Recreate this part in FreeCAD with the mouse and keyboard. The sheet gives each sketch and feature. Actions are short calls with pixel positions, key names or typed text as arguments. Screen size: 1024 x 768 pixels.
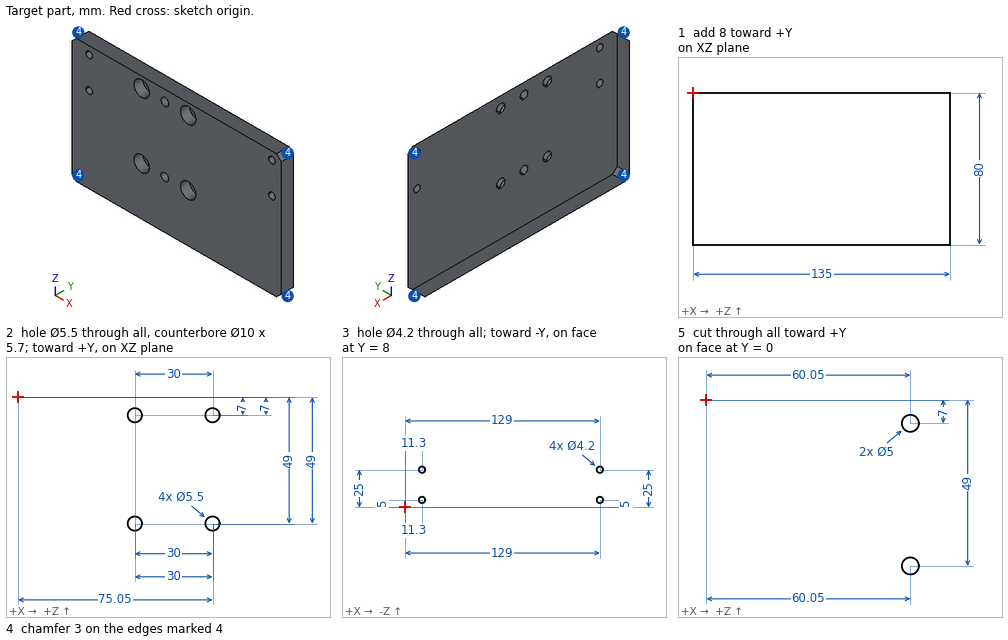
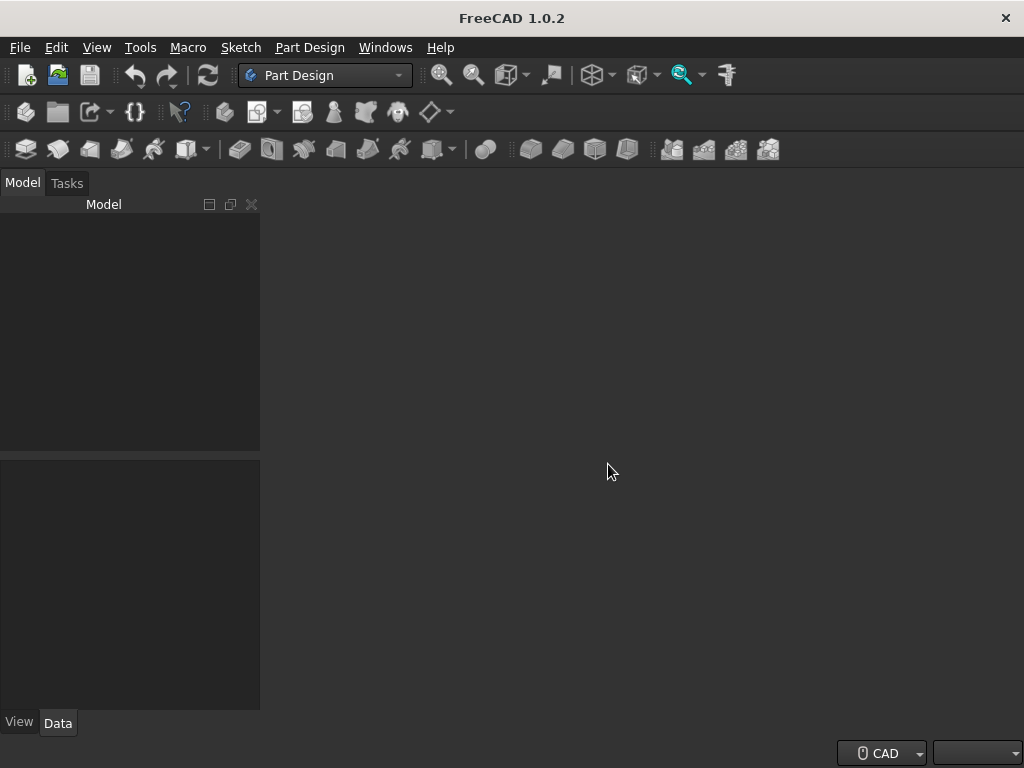
key(ctrl+n)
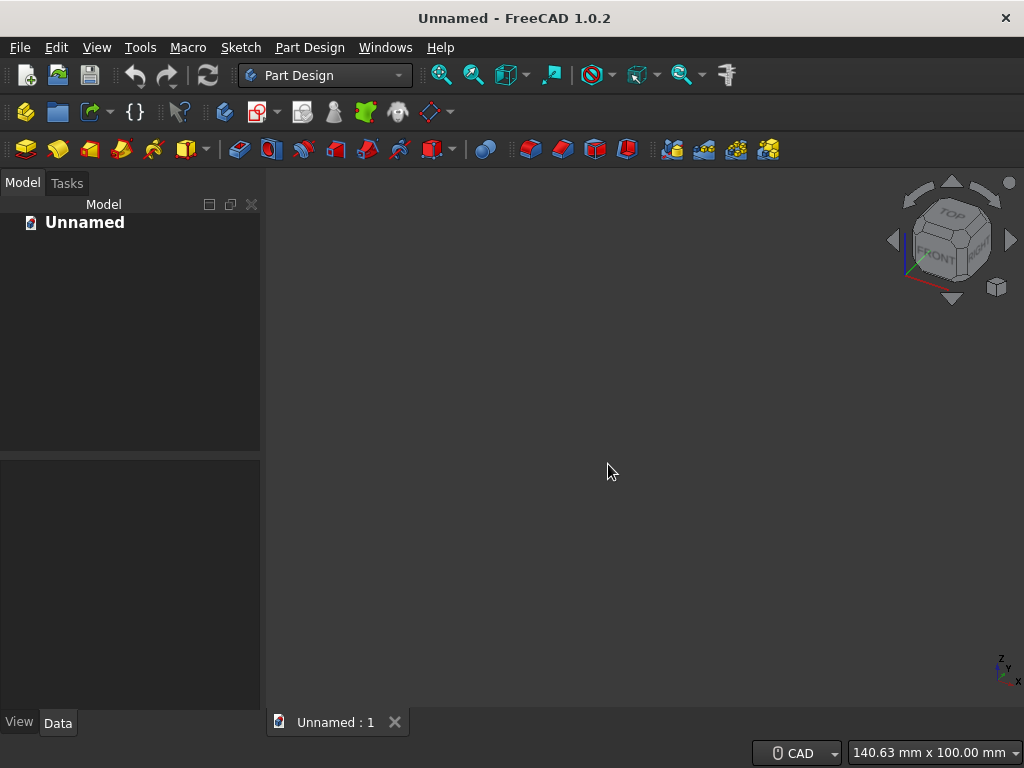
click(258, 112)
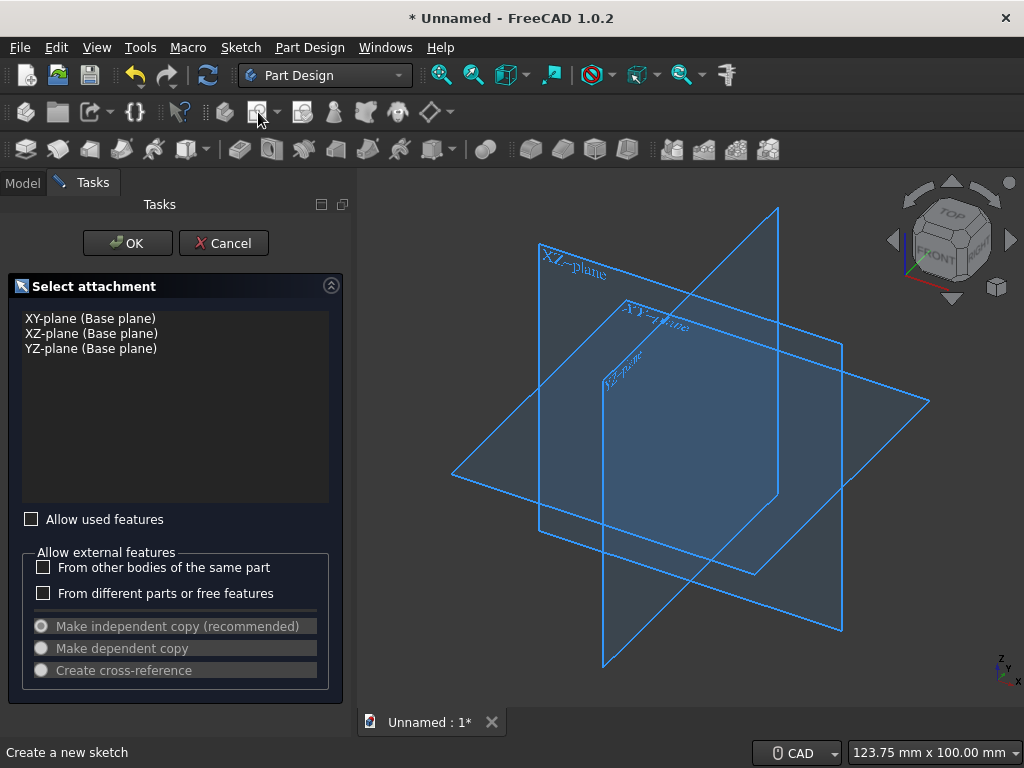
click(82, 334)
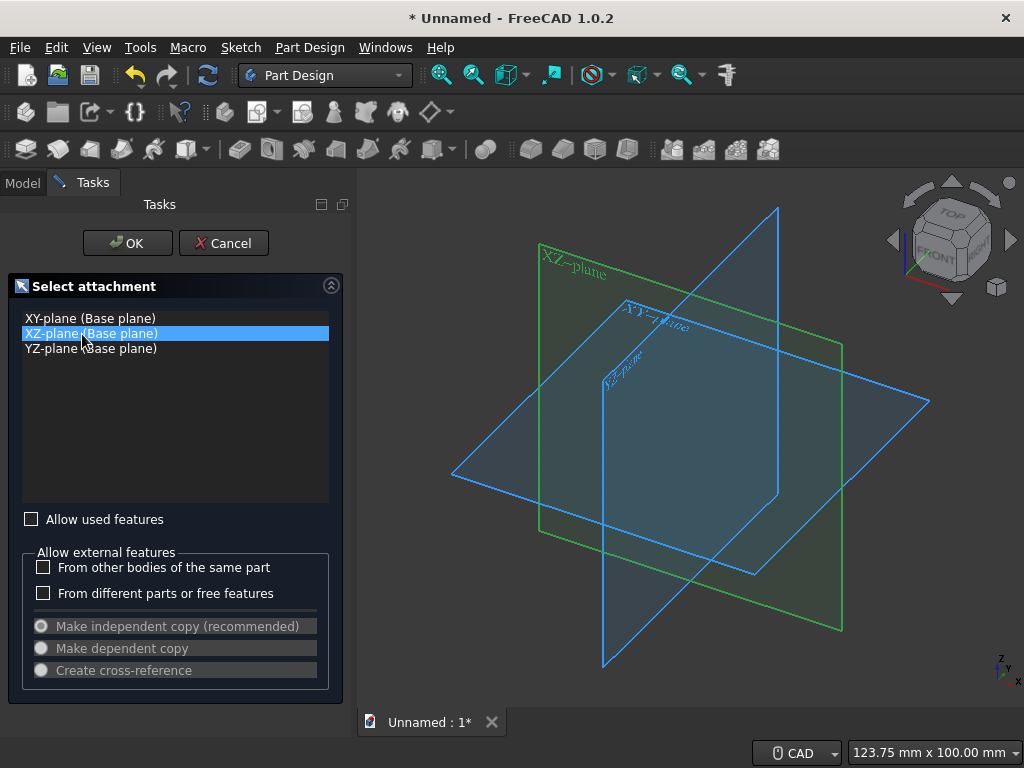
click(128, 243)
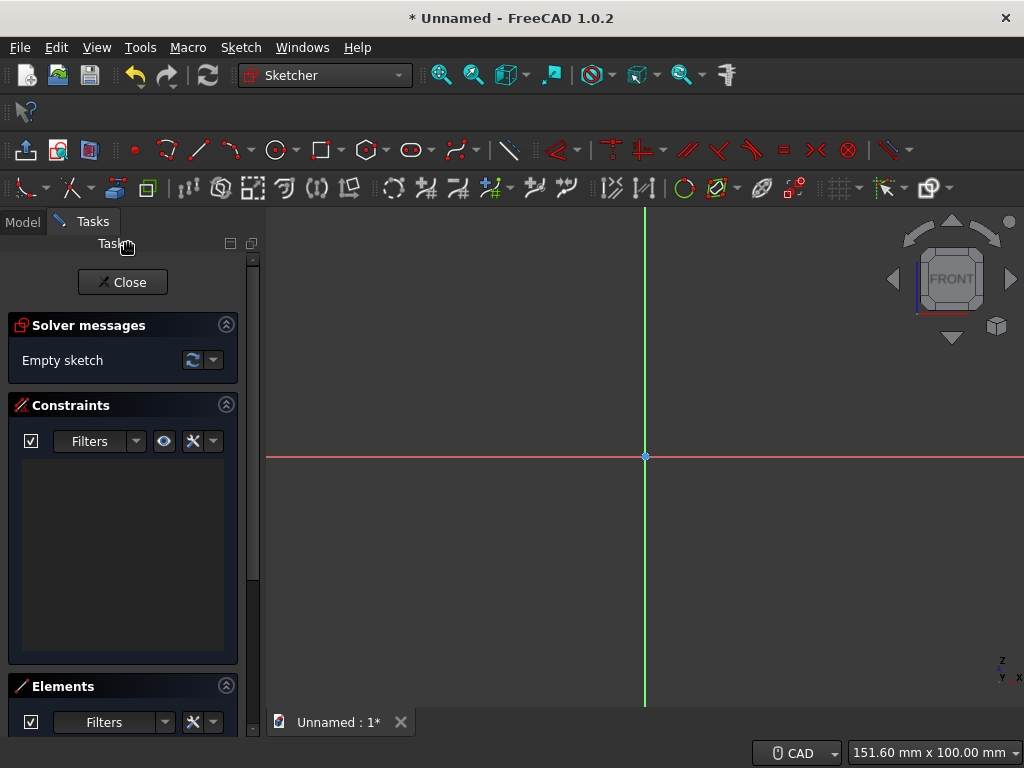
scroll(294, 294, down, 4)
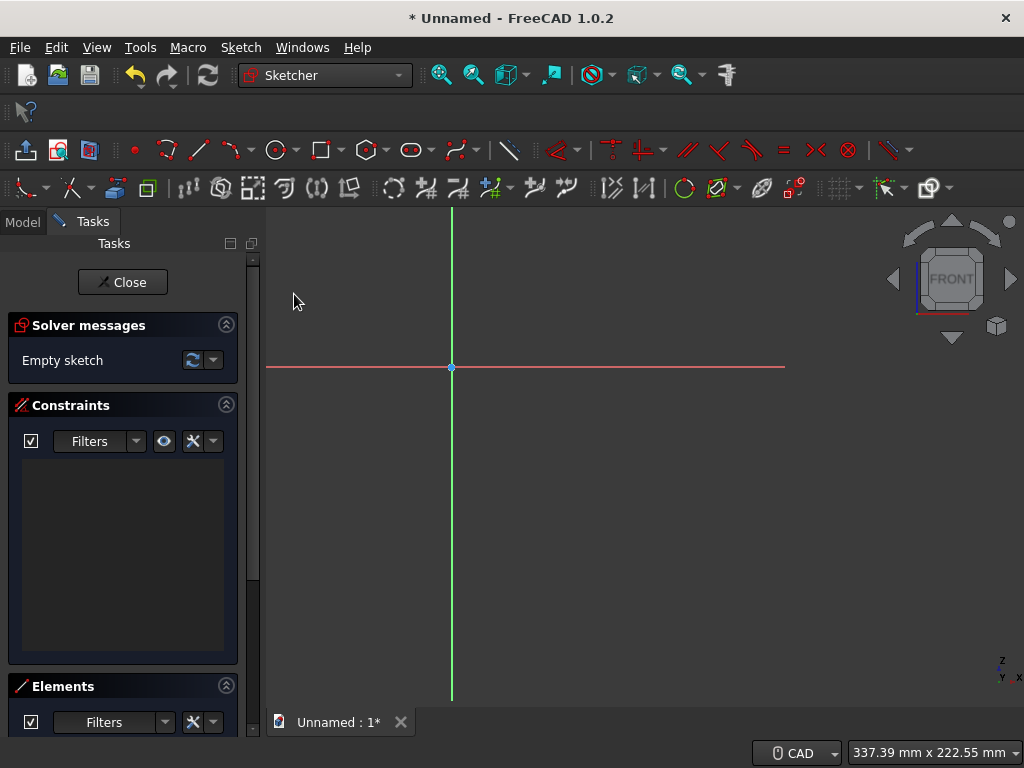
click(322, 150)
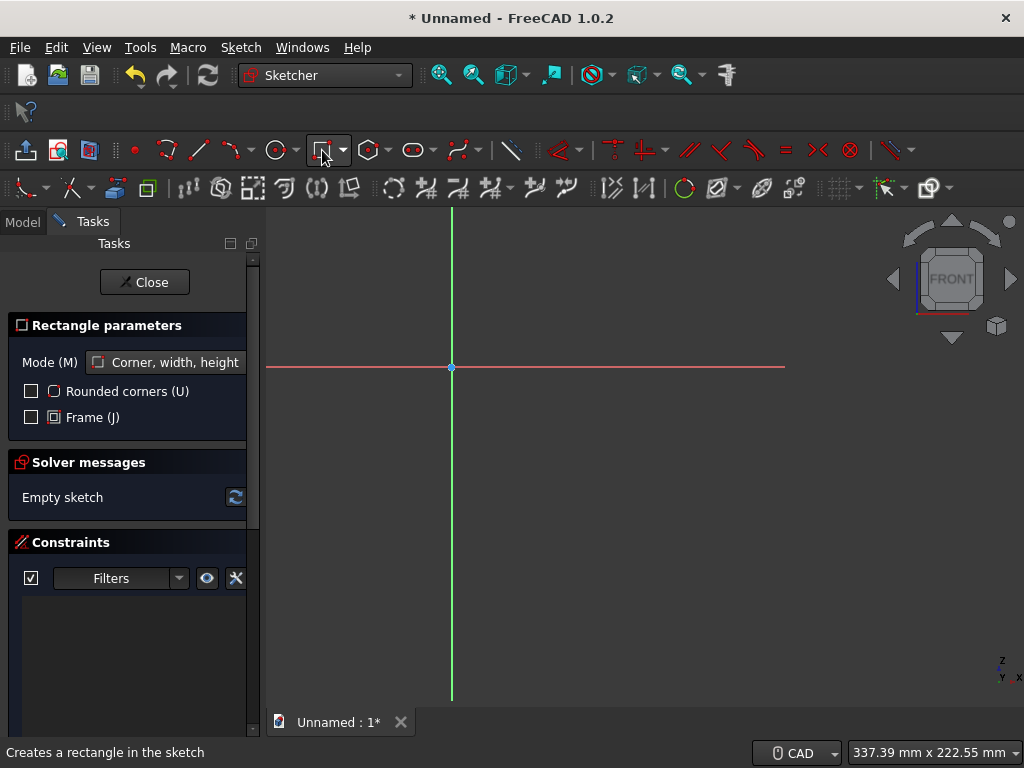
click(452, 367)
move(755, 547)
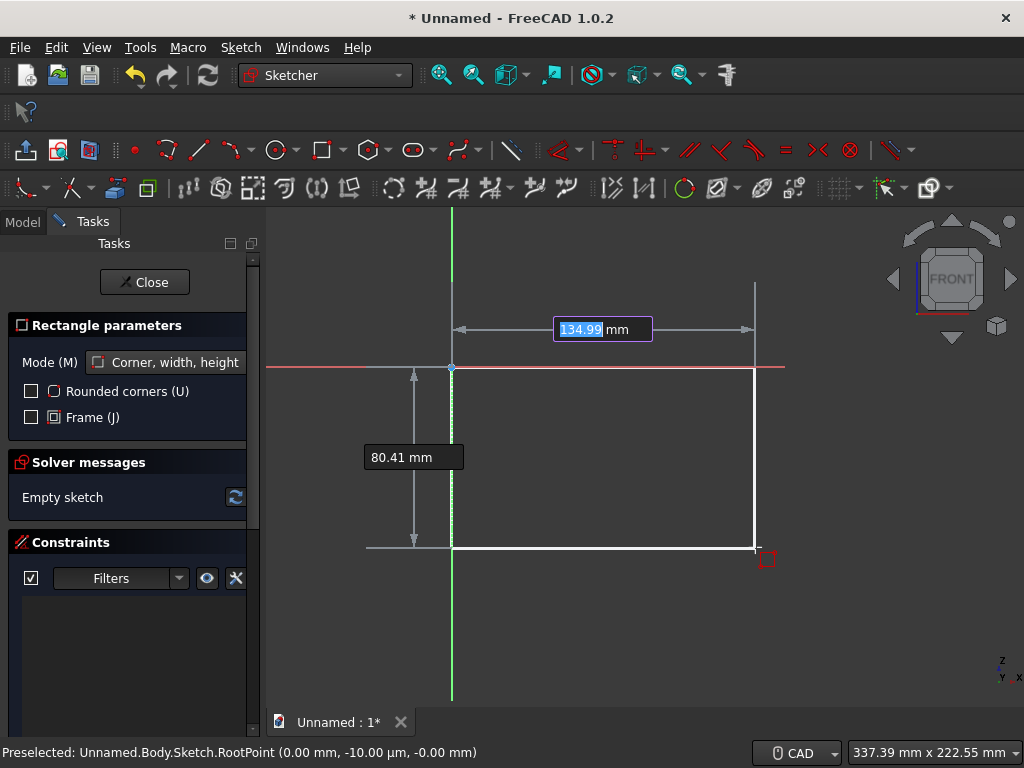
text(135)
key(Tab)
text(80)
key(Return)
key(Escape)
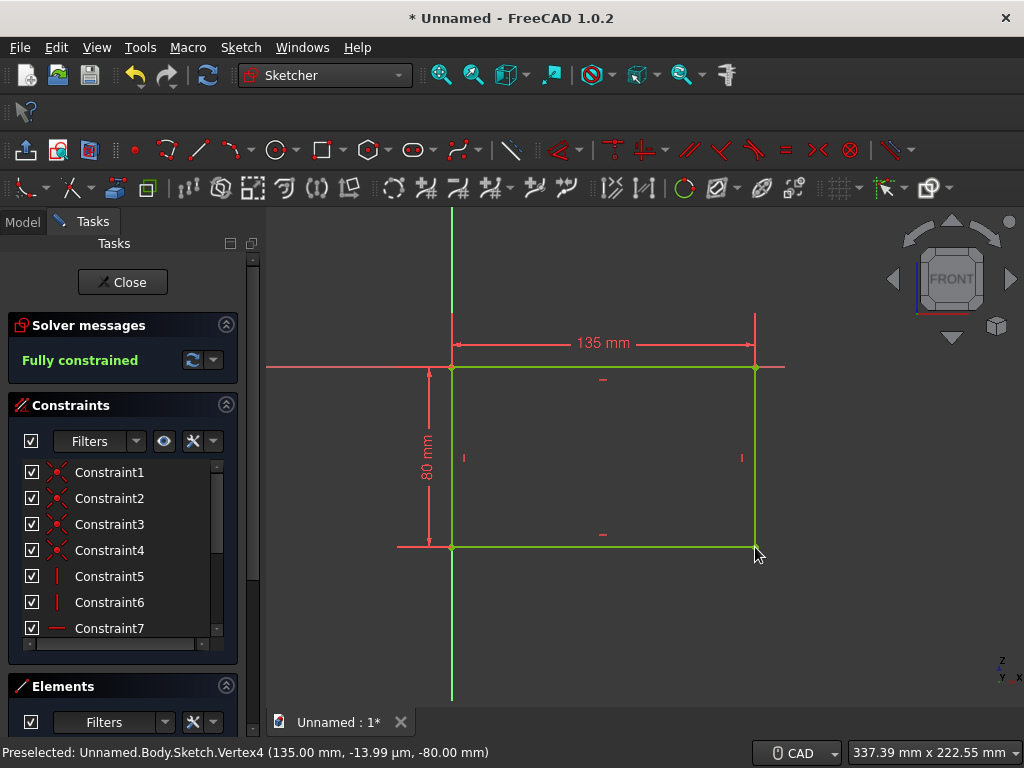
click(123, 282)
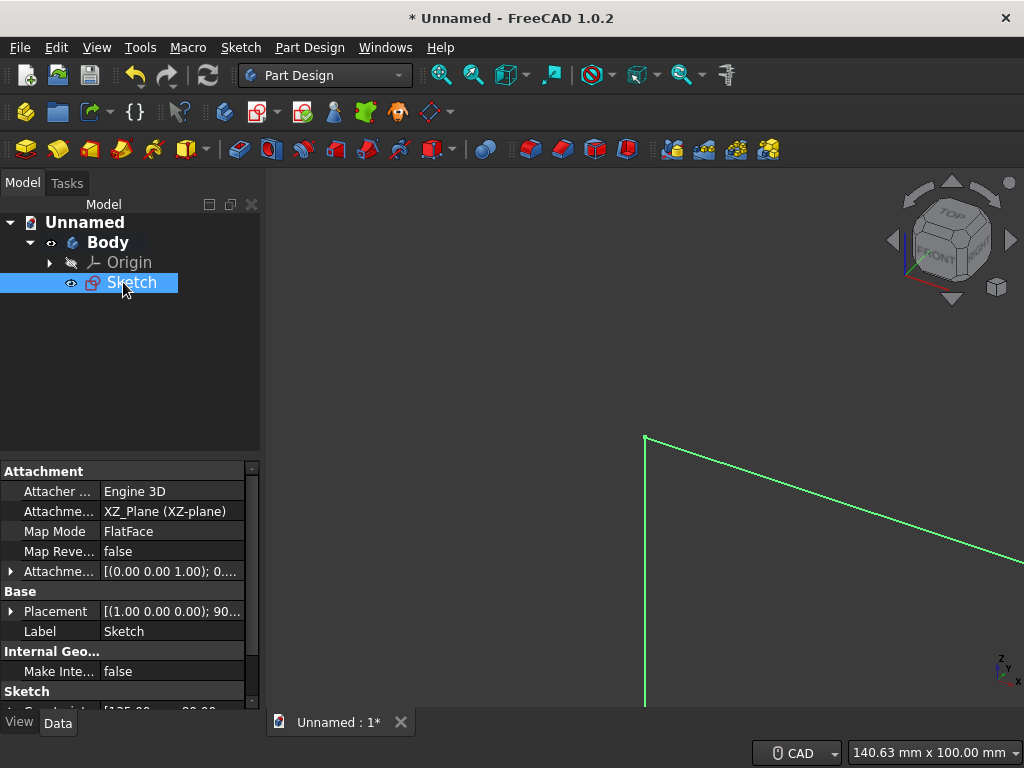
click(26, 150)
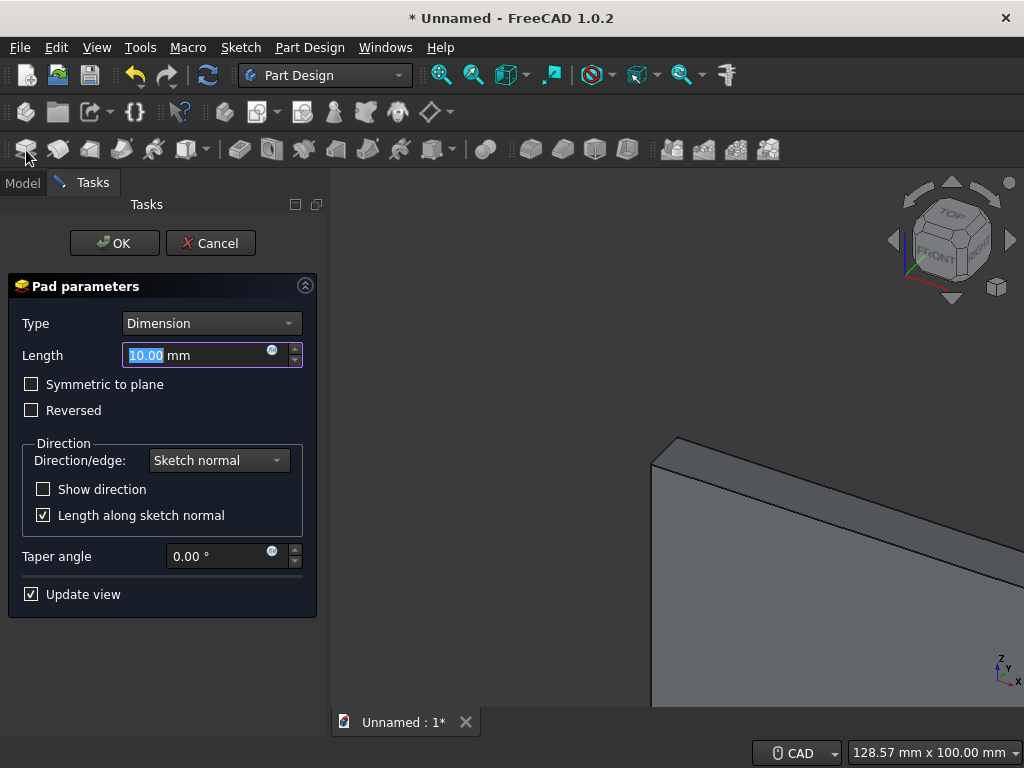
text(8)
key(Tab)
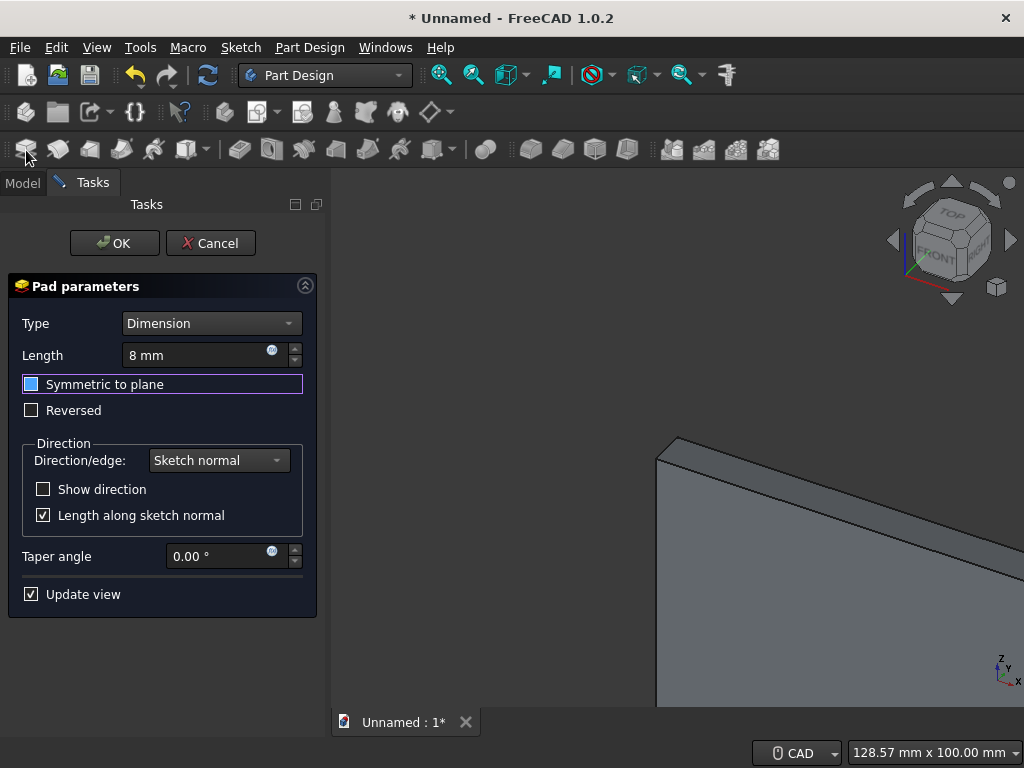
click(30, 410)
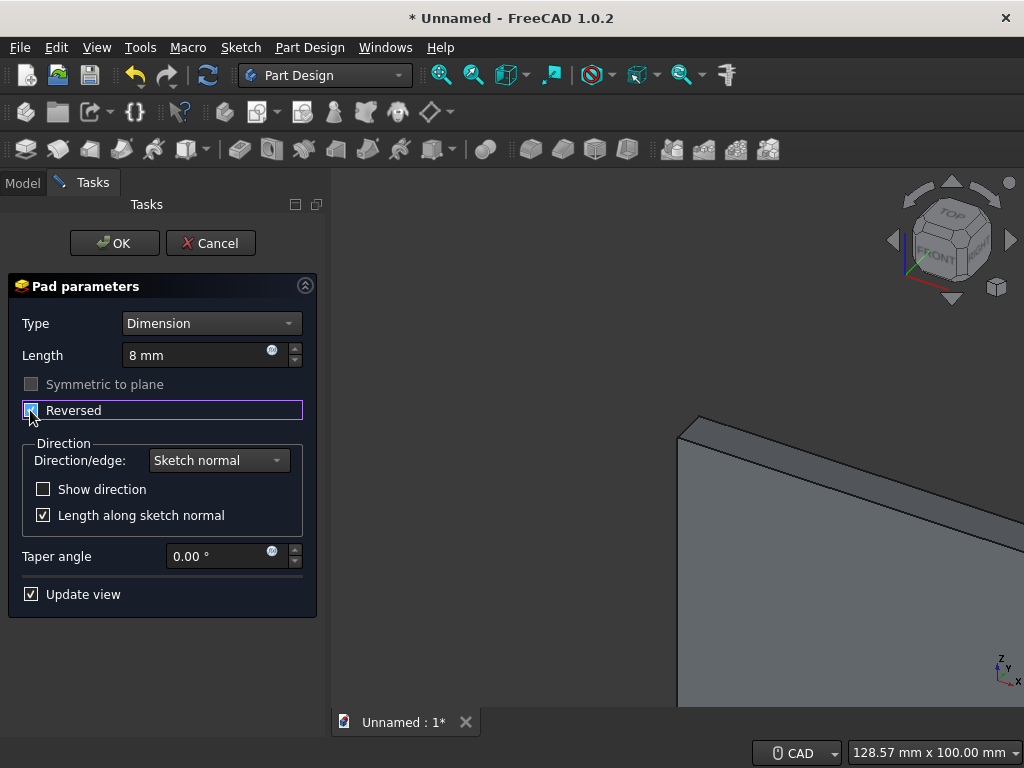
click(115, 243)